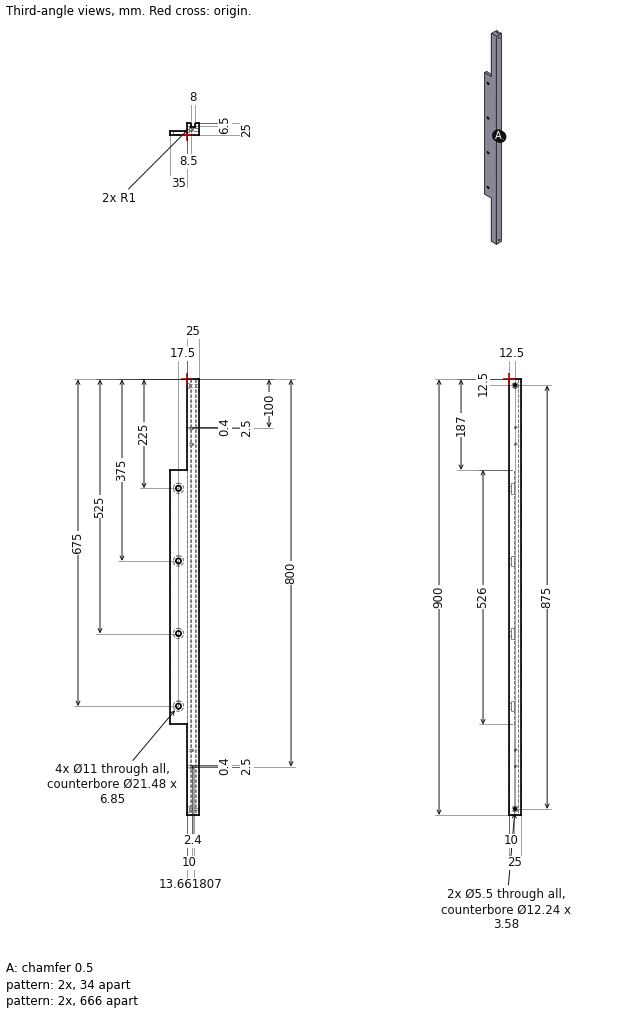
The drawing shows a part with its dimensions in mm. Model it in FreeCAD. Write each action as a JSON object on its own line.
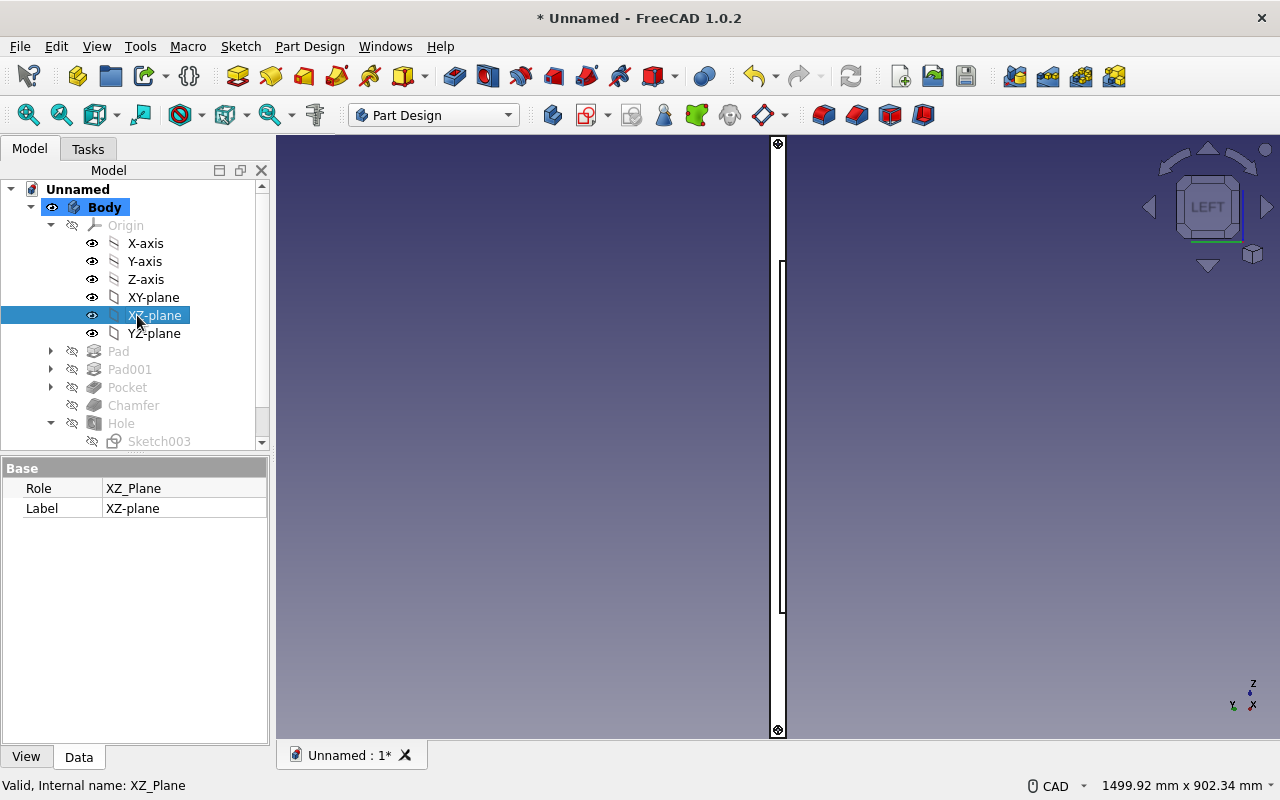
{"action": "left_click", "coordinate": [762, 116]}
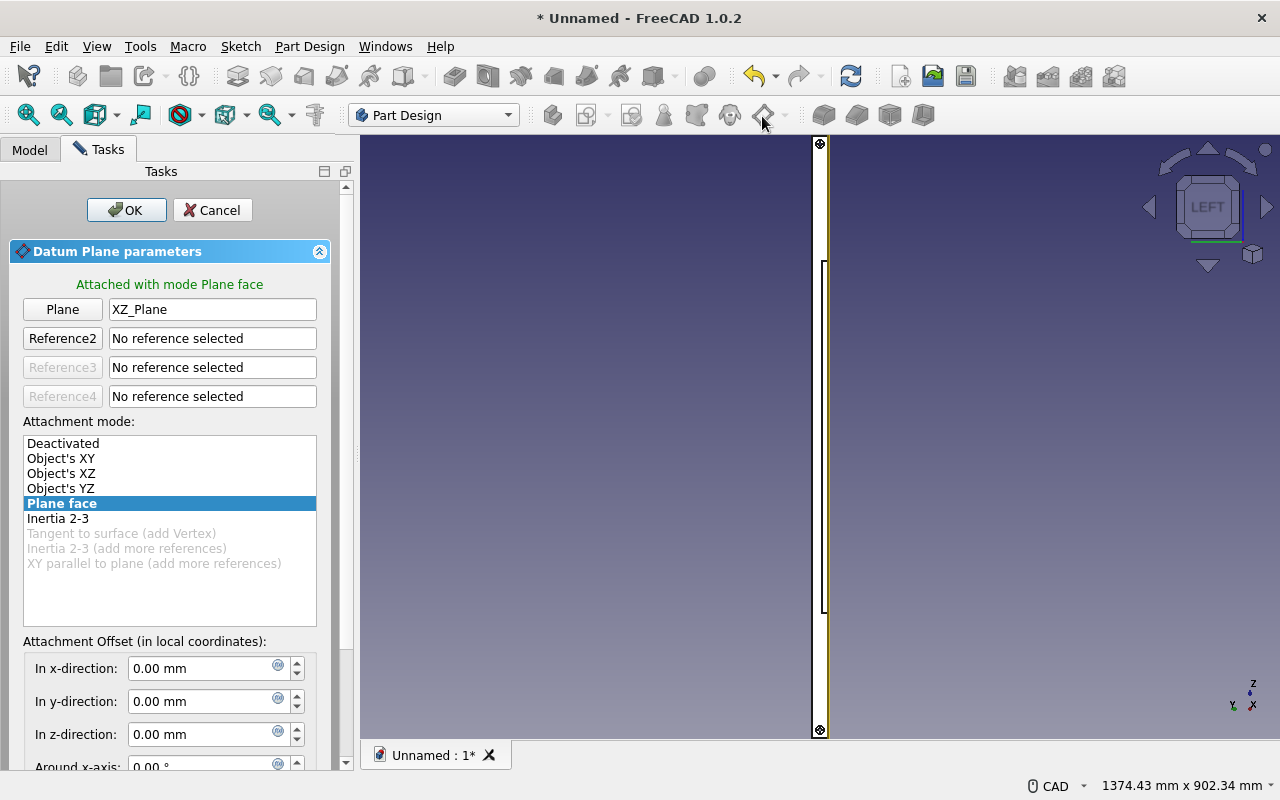
{"action": "triple_click", "coordinate": [210, 734]}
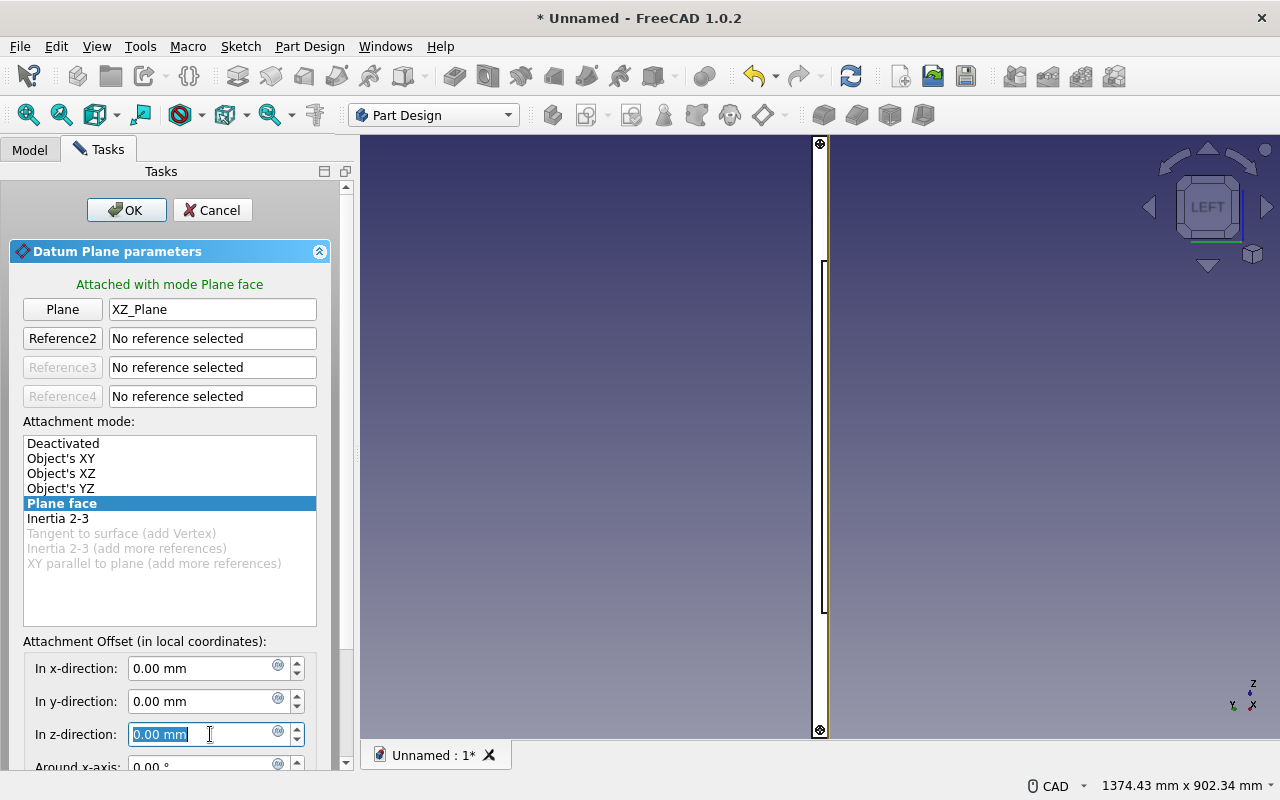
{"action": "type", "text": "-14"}
{"action": "key", "text": "Tab"}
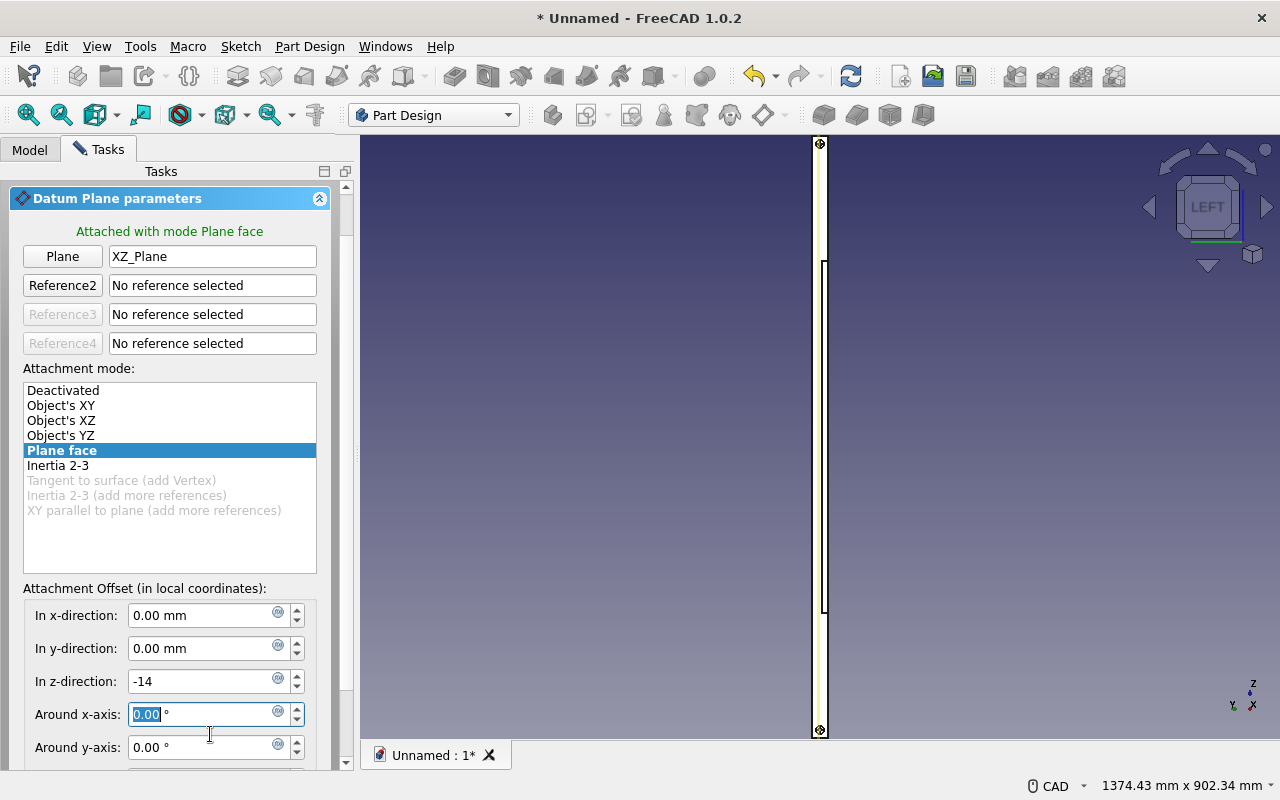
{"action": "scroll", "coordinate": [346, 476], "scroll_direction": "up", "scroll_amount": 2}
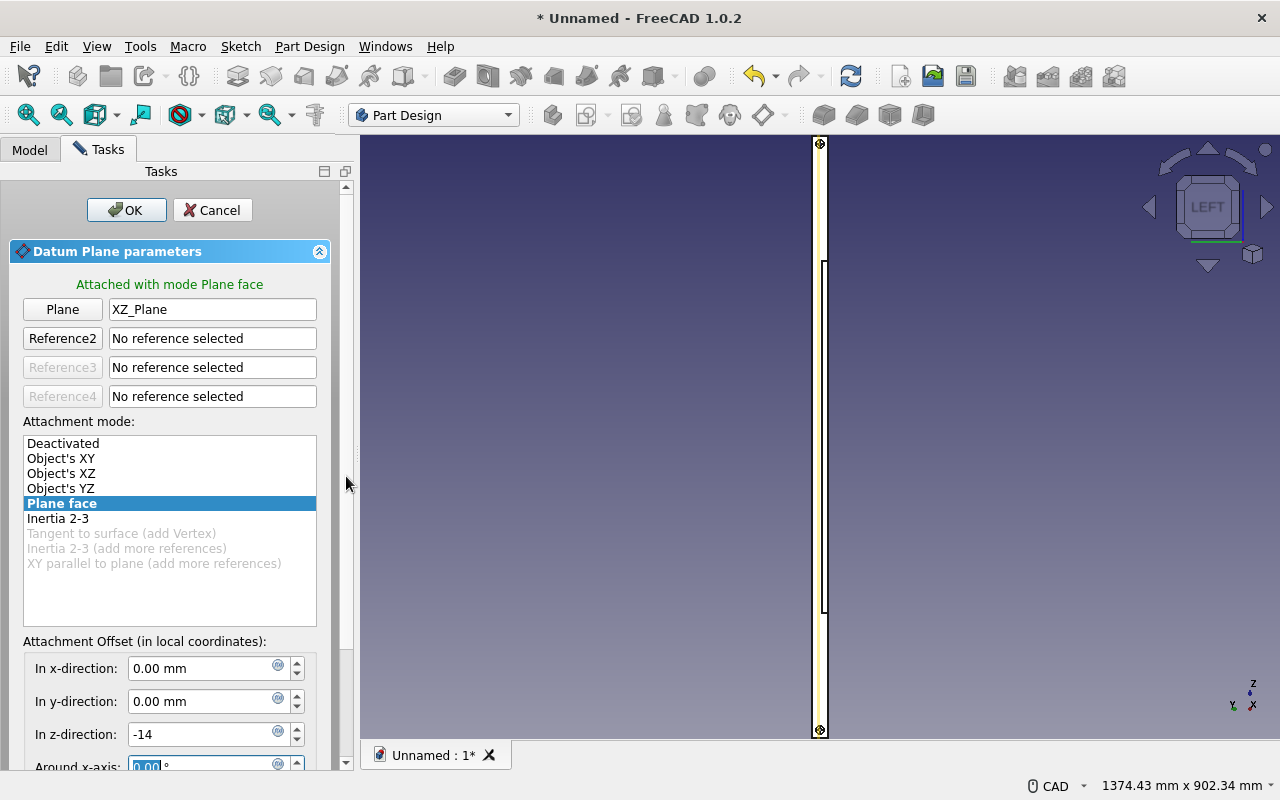
{"action": "left_click", "coordinate": [127, 210]}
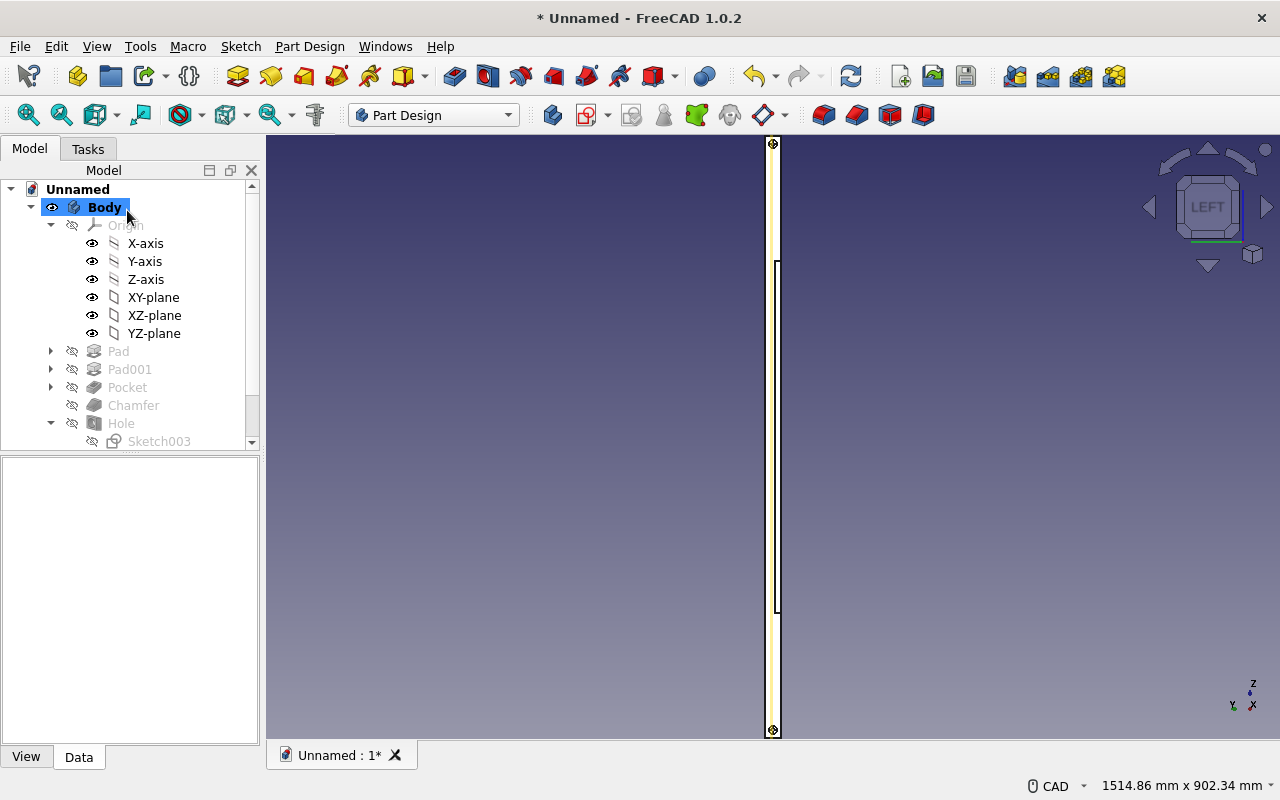
{"action": "scroll", "coordinate": [101, 311], "scroll_direction": "down", "scroll_amount": 3}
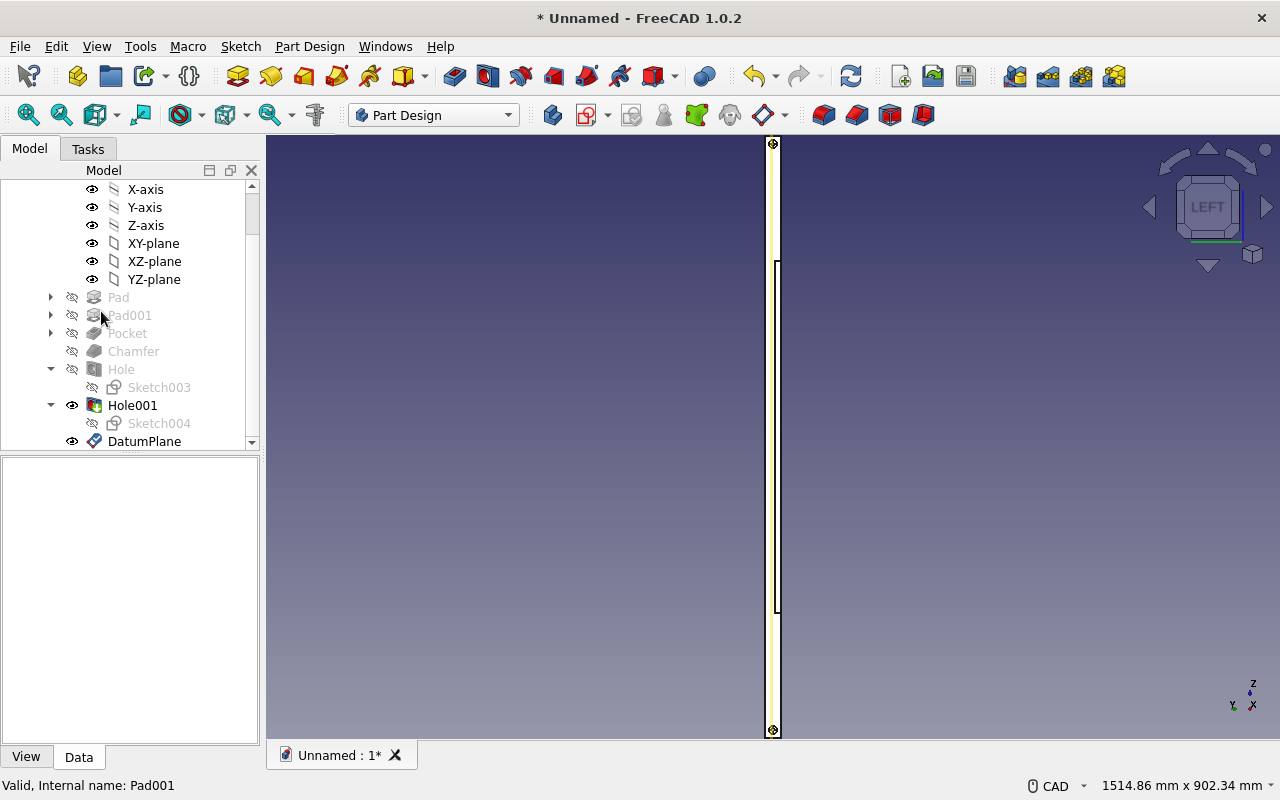
{"action": "left_click", "coordinate": [117, 441]}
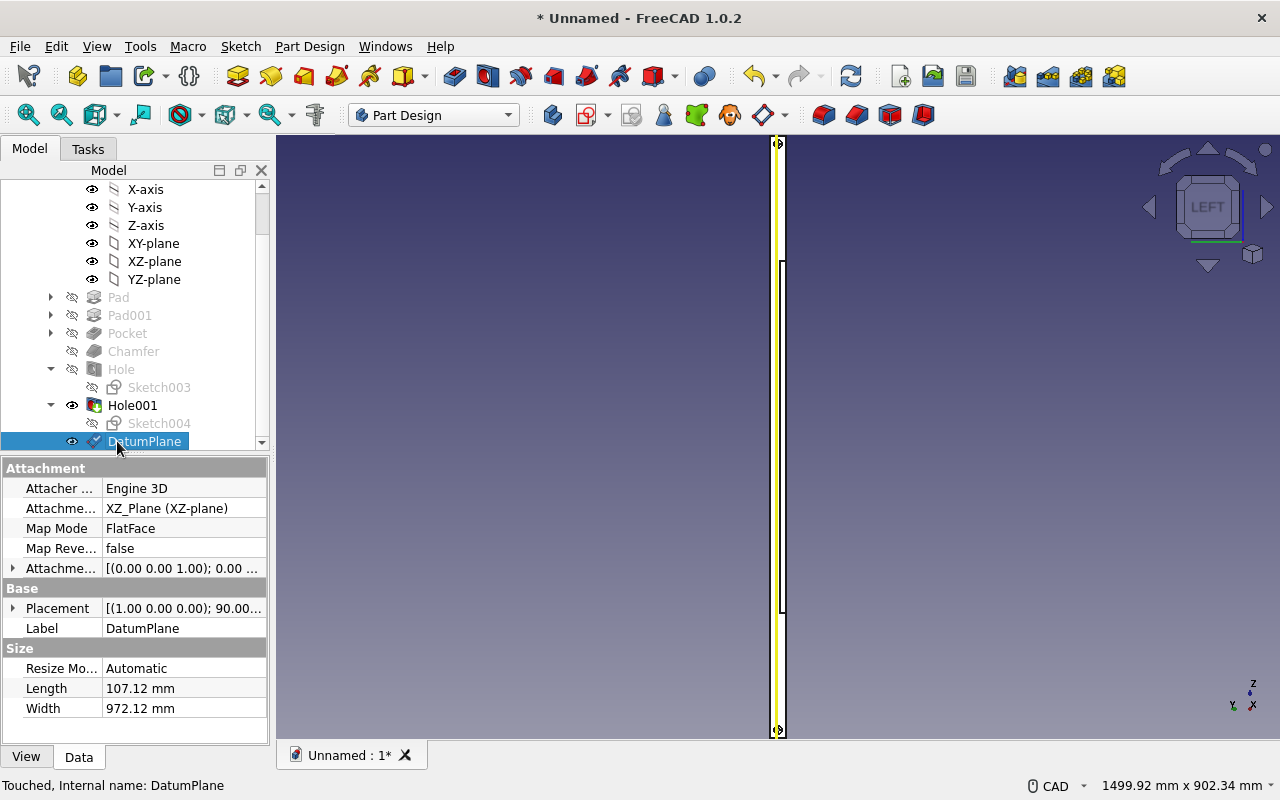
{"action": "left_click", "coordinate": [586, 116]}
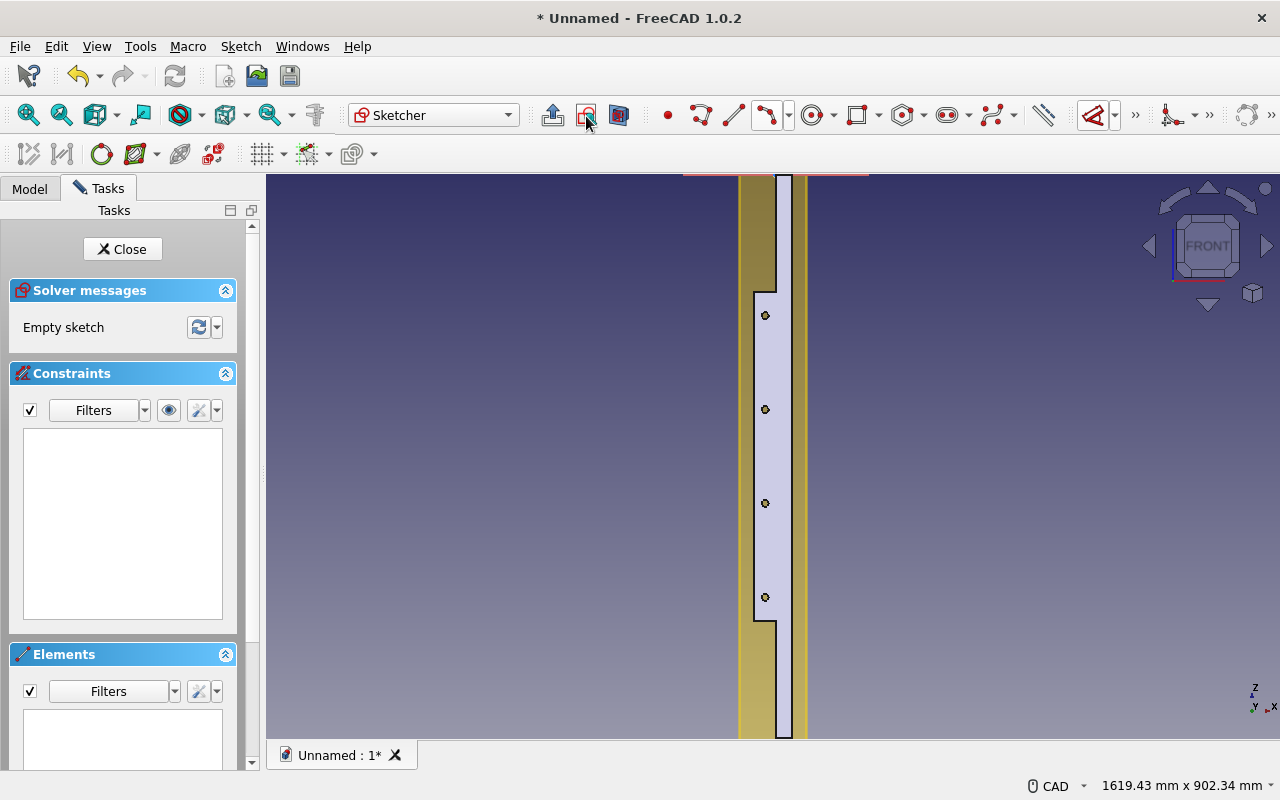
{"action": "left_click", "coordinate": [619, 116]}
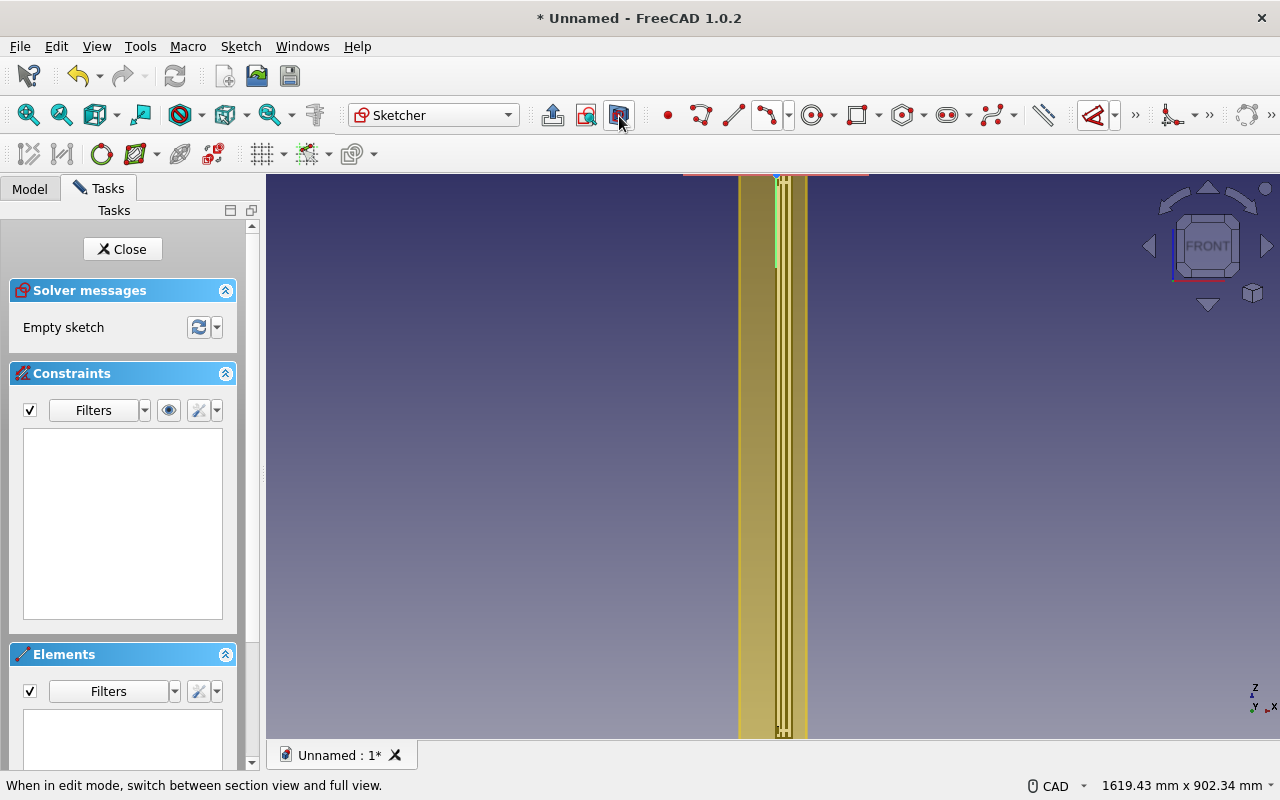
{"action": "scroll", "coordinate": [786, 686], "scroll_direction": "up", "scroll_amount": 15}